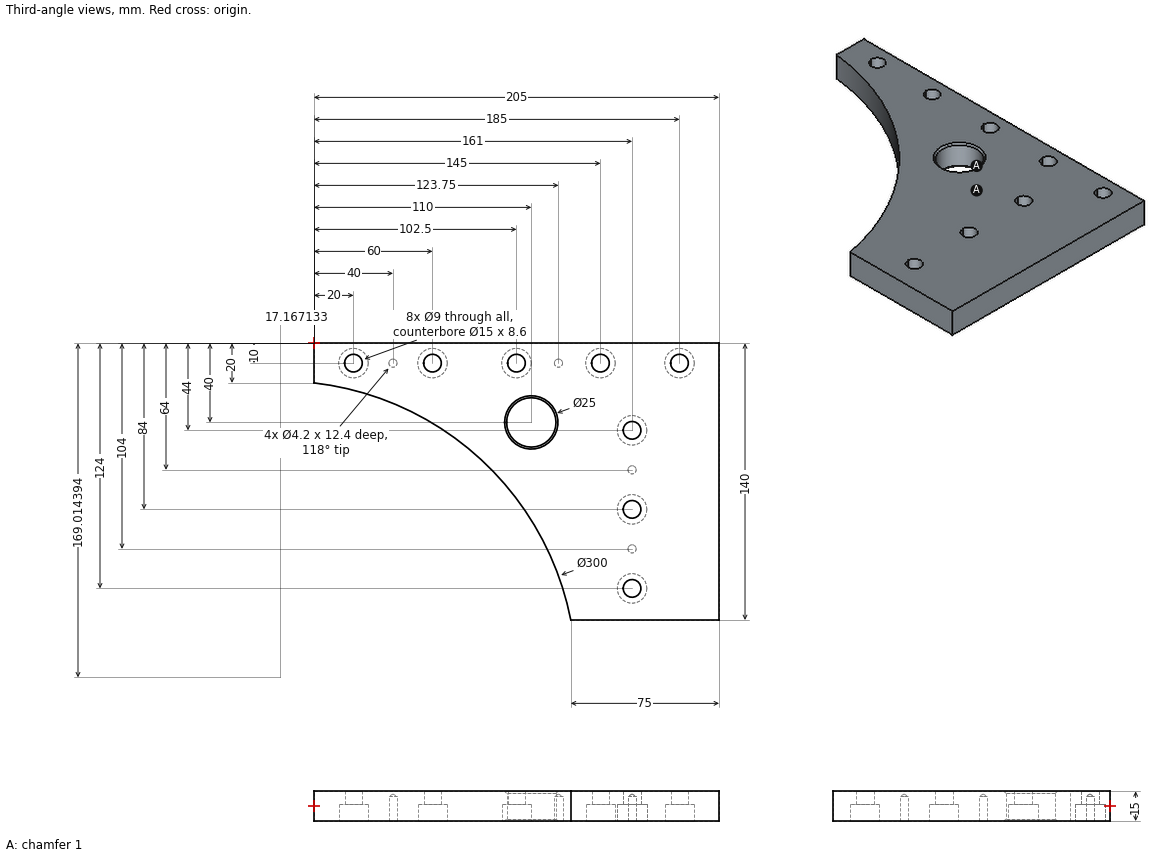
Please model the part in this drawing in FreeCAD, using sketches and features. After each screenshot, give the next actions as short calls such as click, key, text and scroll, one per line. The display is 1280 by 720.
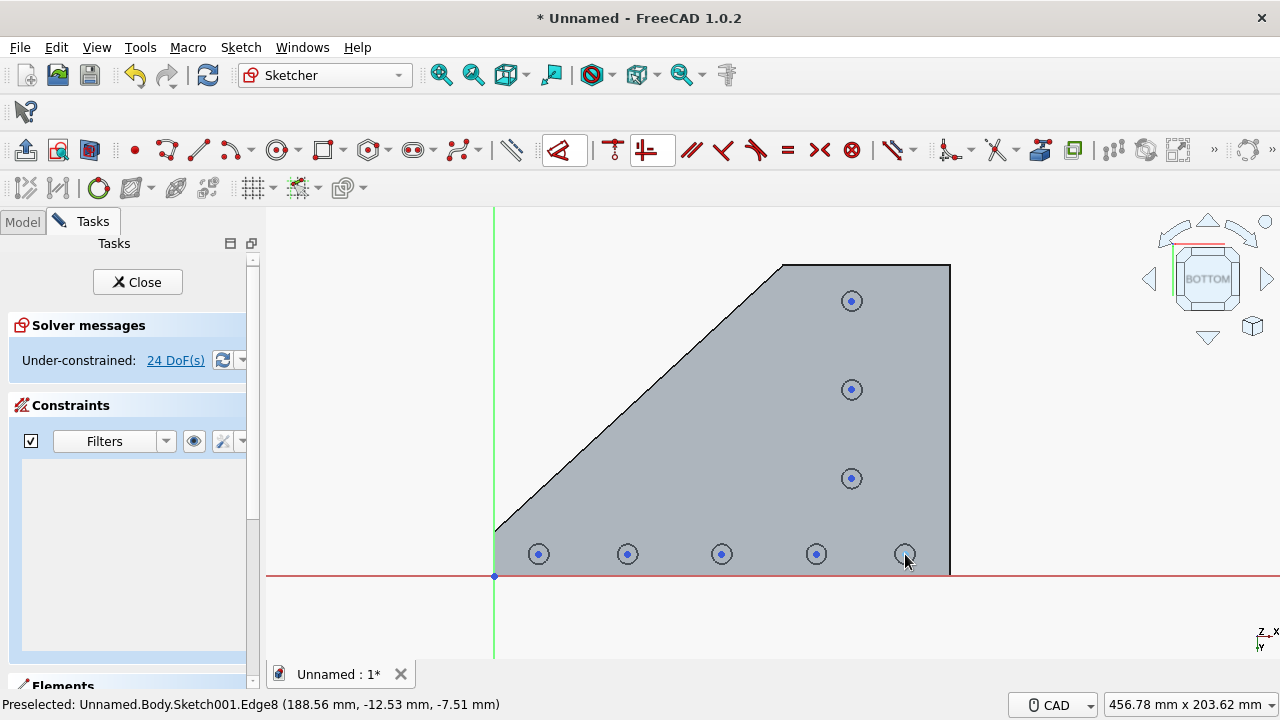
scroll(546, 547, up, 2)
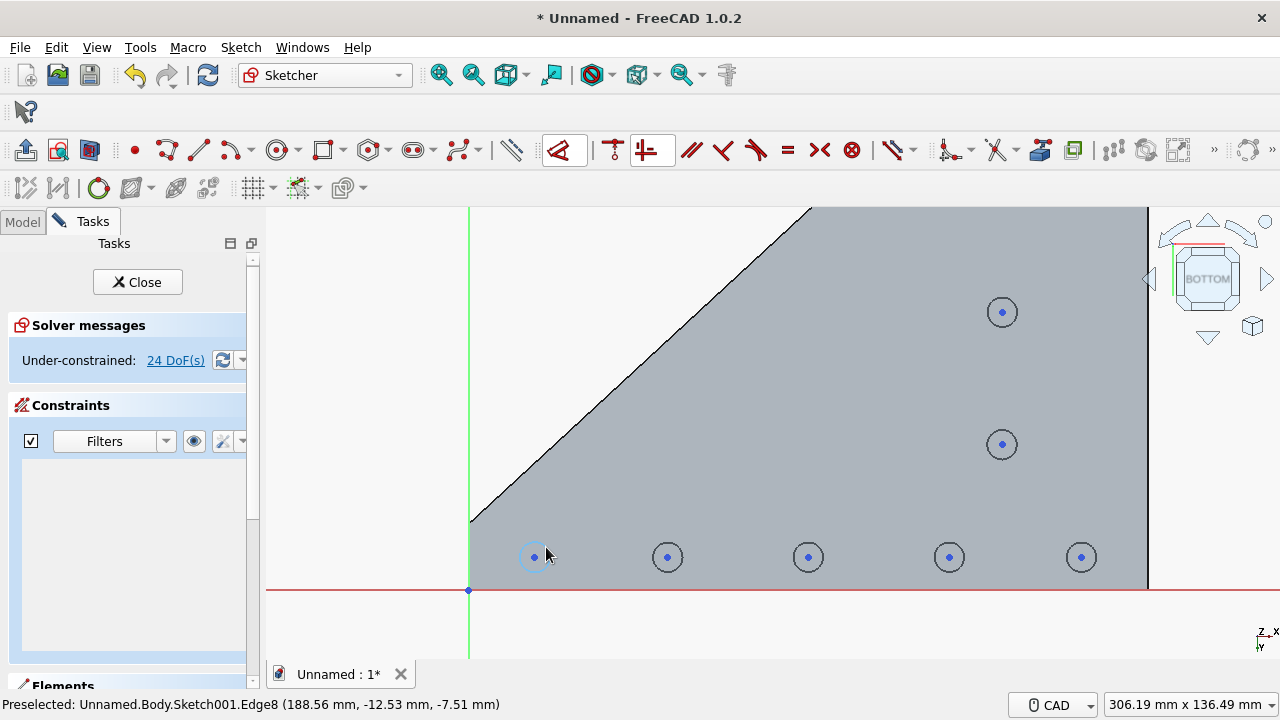
click(546, 547)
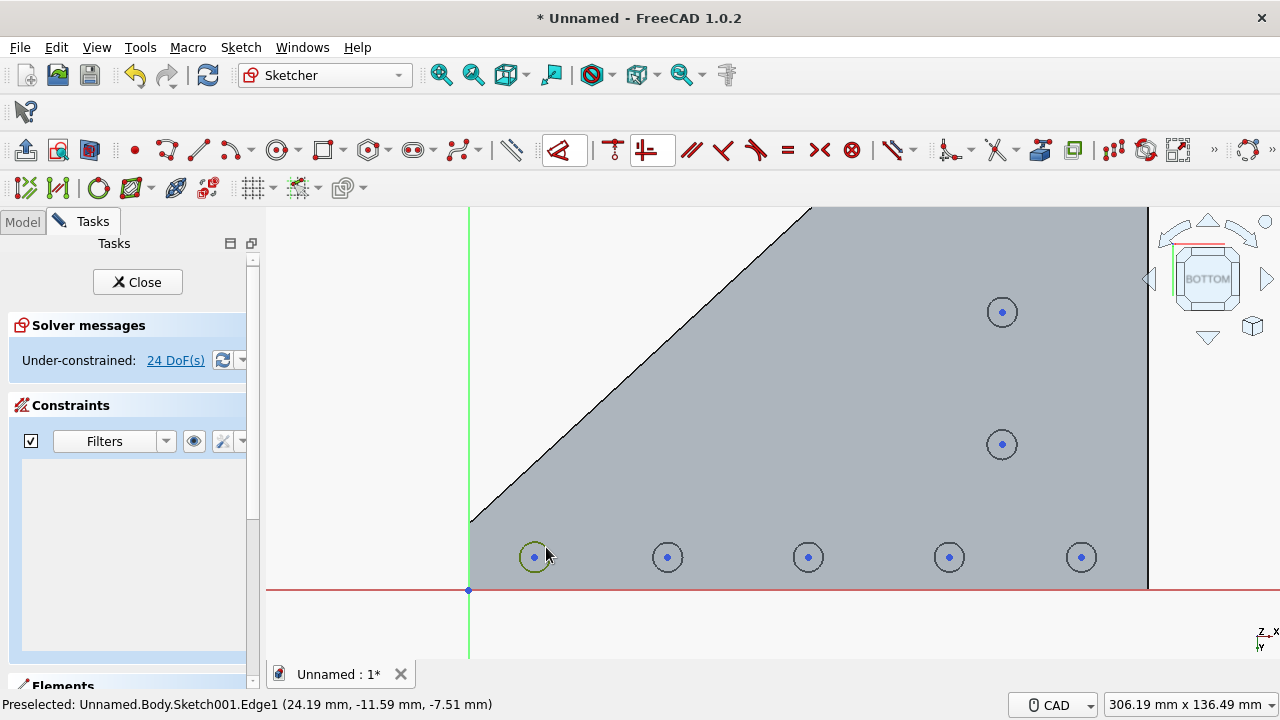
click(678, 547)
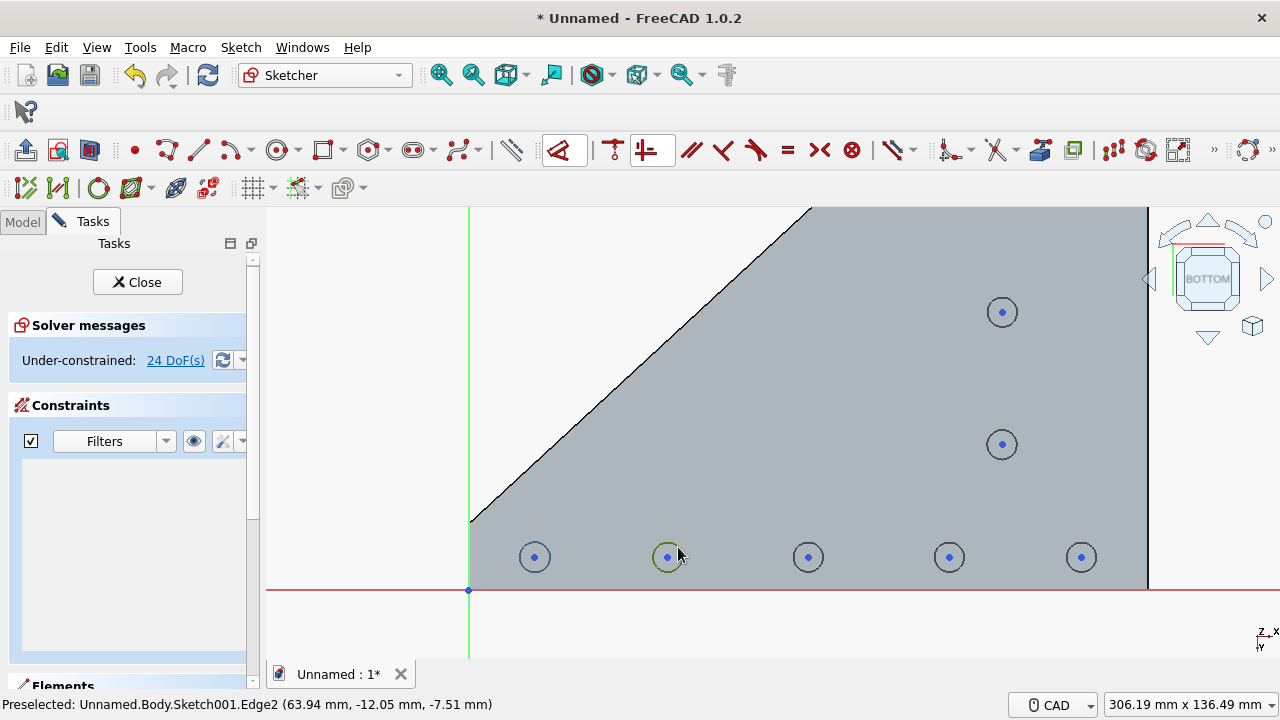
click(819, 547)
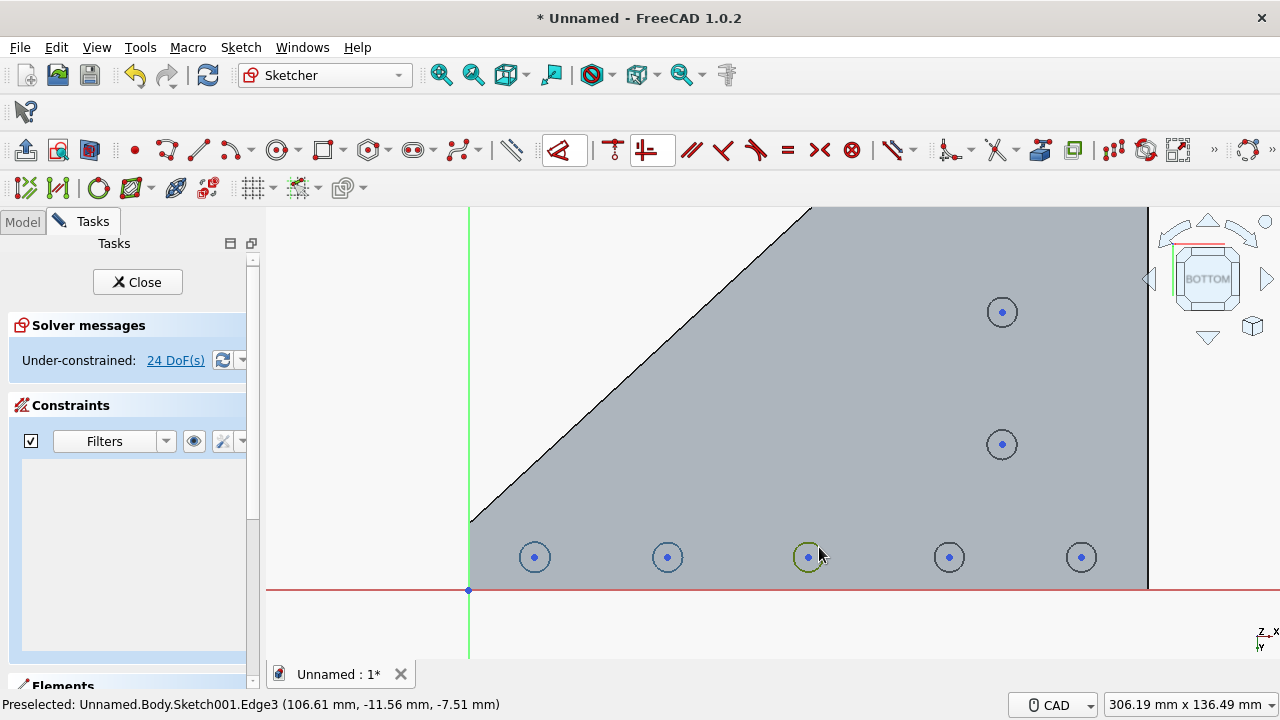
click(960, 547)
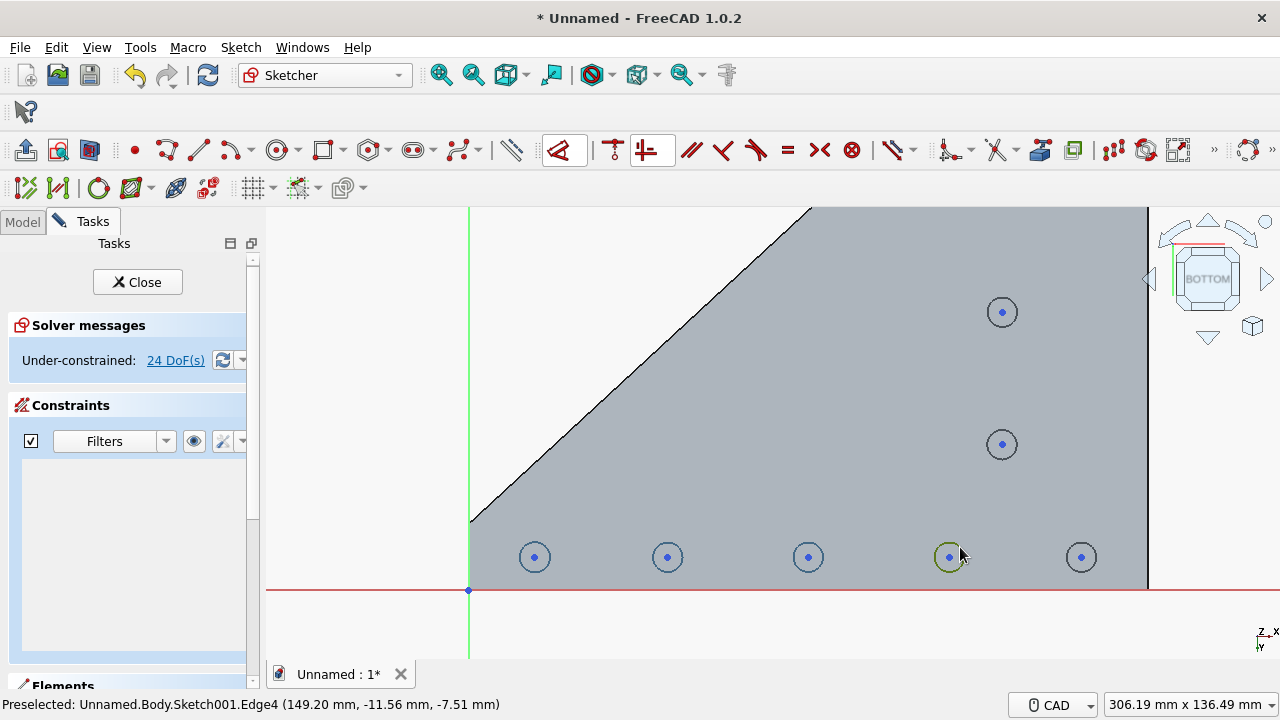
click(1012, 434)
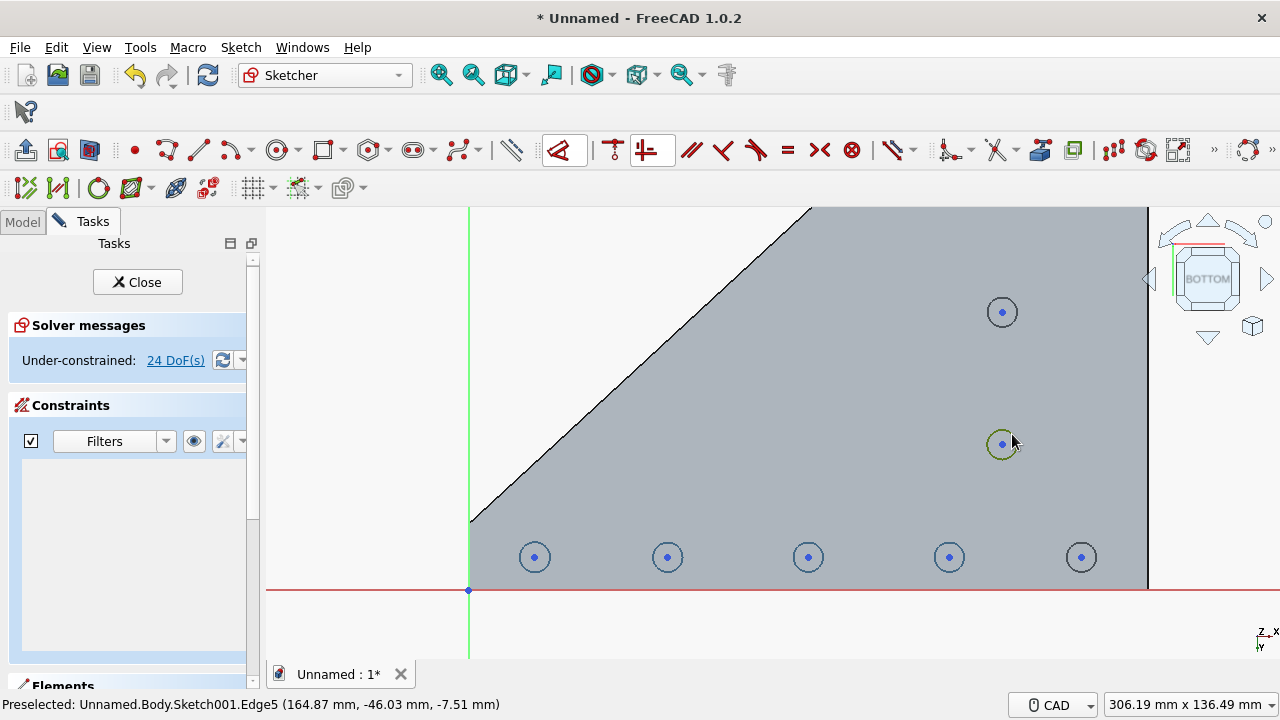
click(1013, 302)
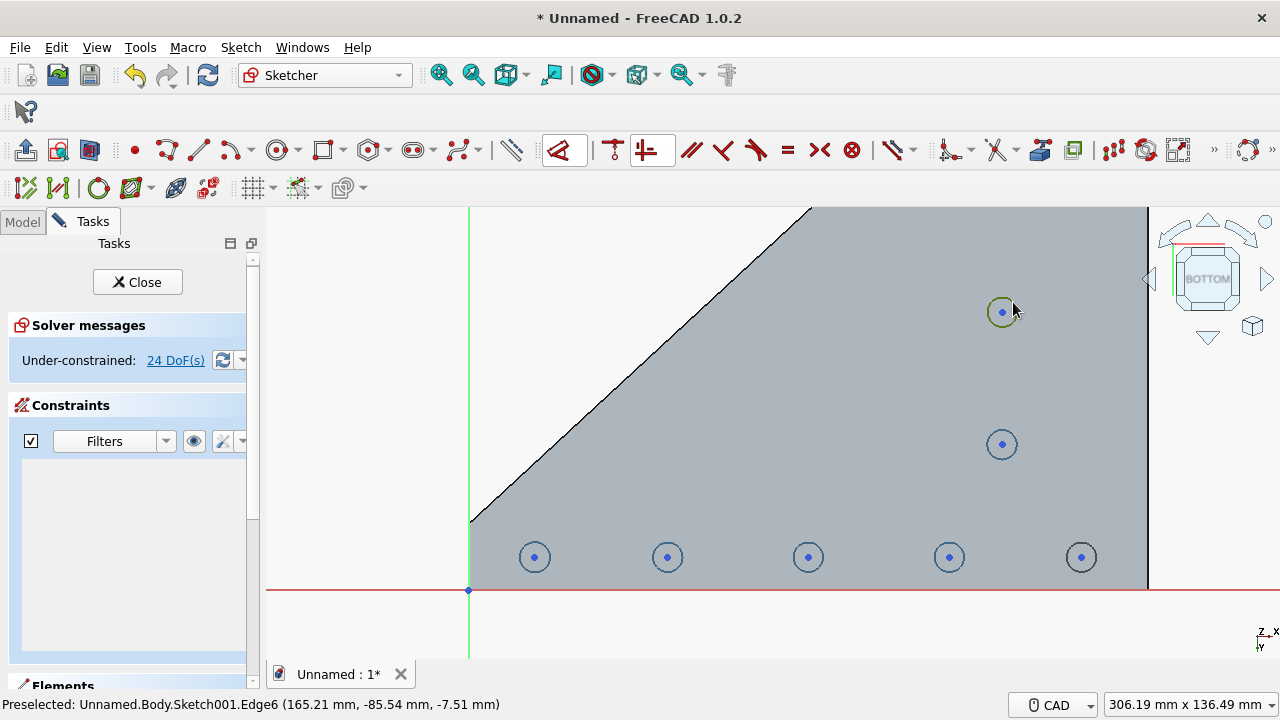
scroll(545, 546, down, 2)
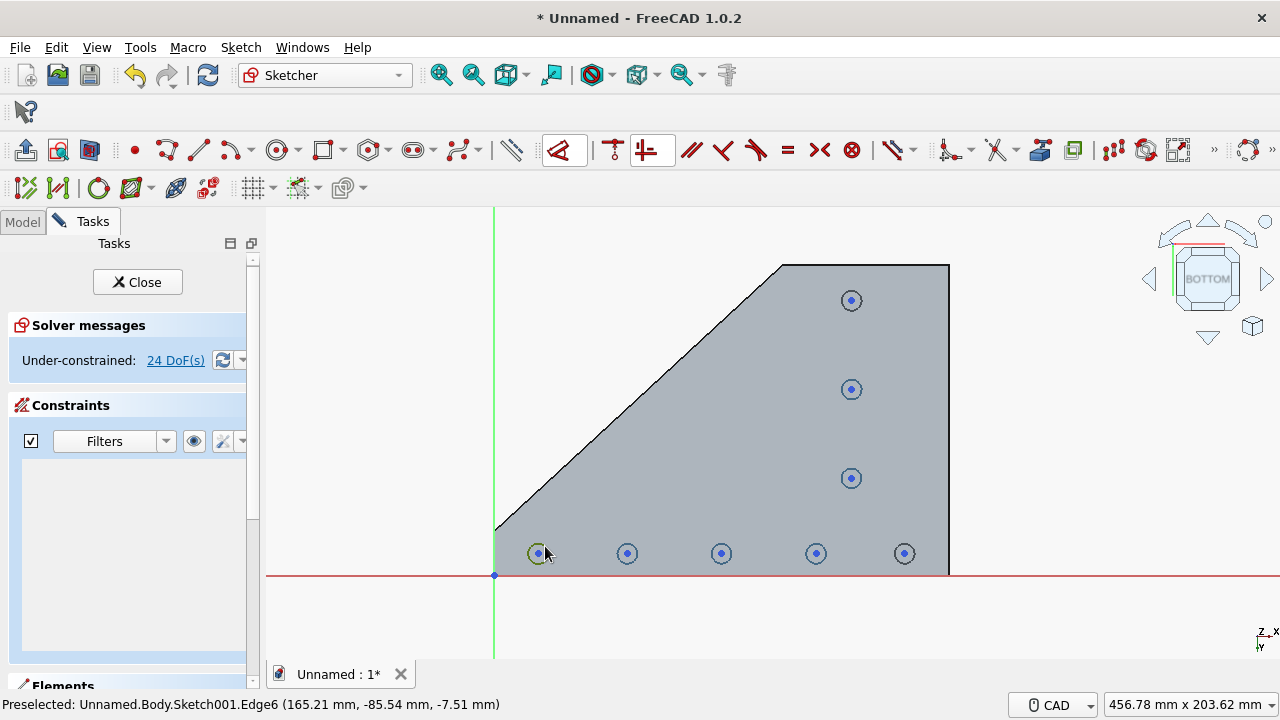
scroll(859, 294, up, 2)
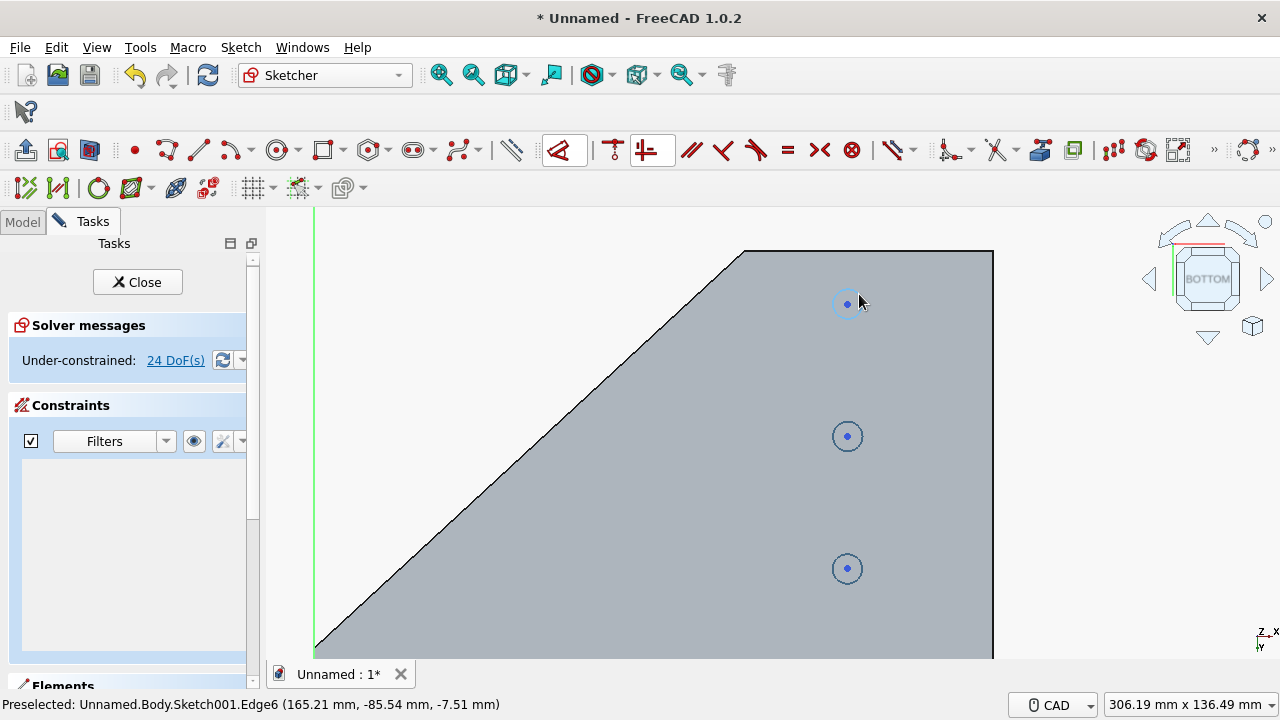
click(858, 294)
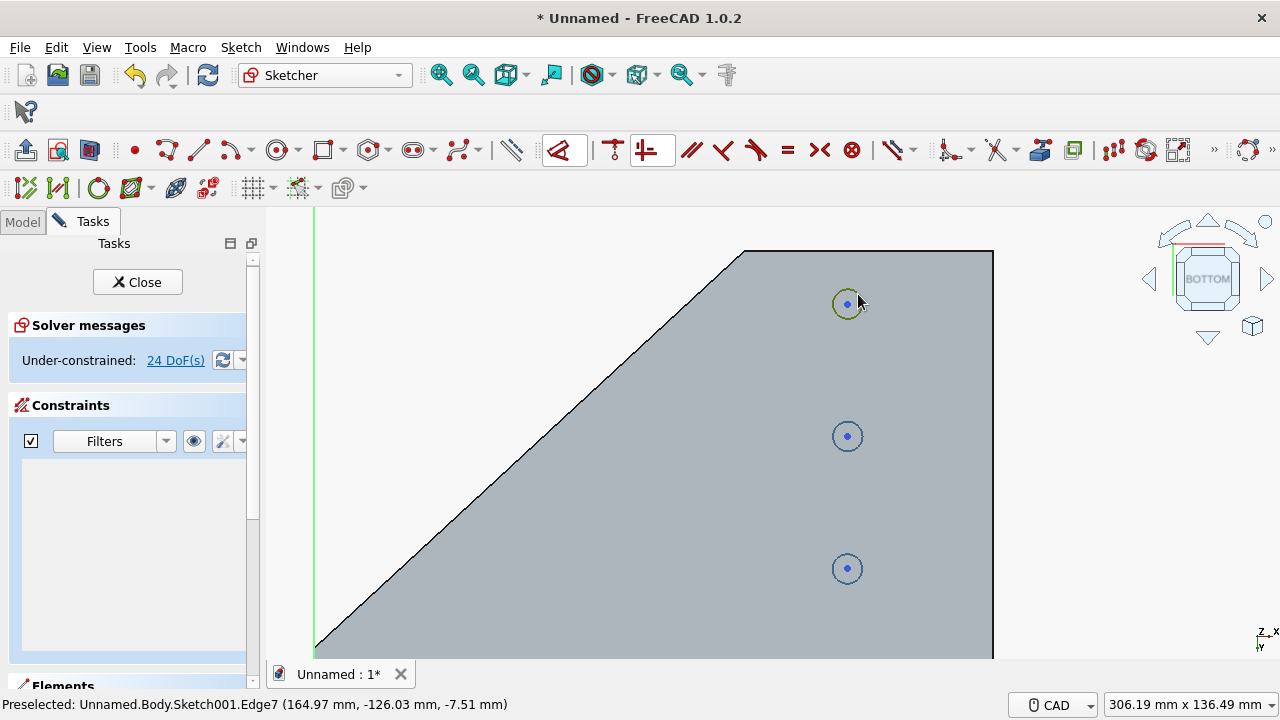
scroll(860, 294, down, 2)